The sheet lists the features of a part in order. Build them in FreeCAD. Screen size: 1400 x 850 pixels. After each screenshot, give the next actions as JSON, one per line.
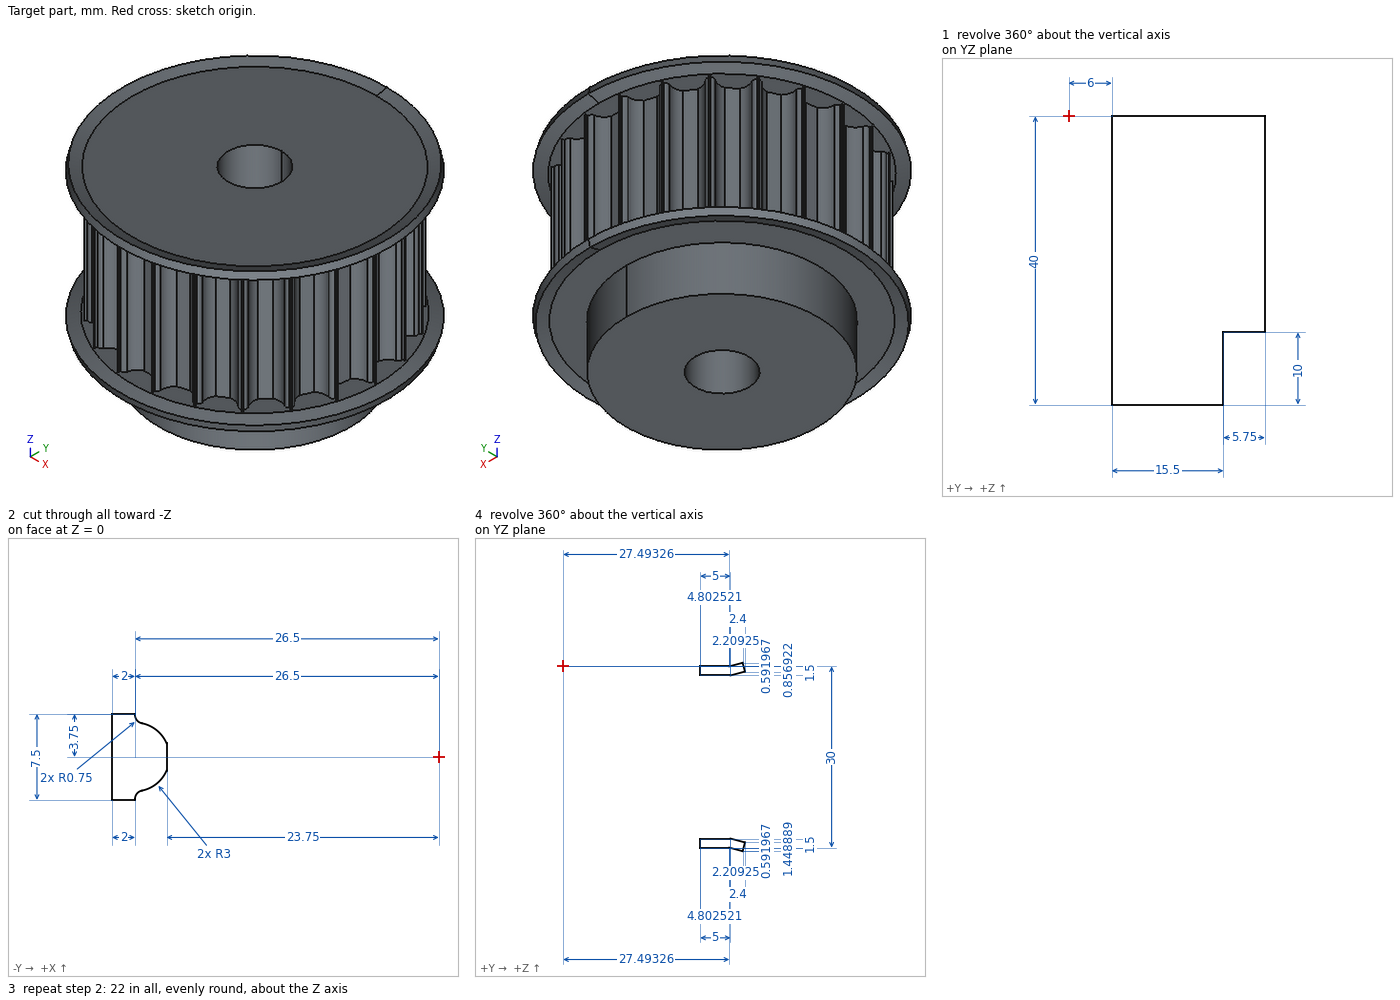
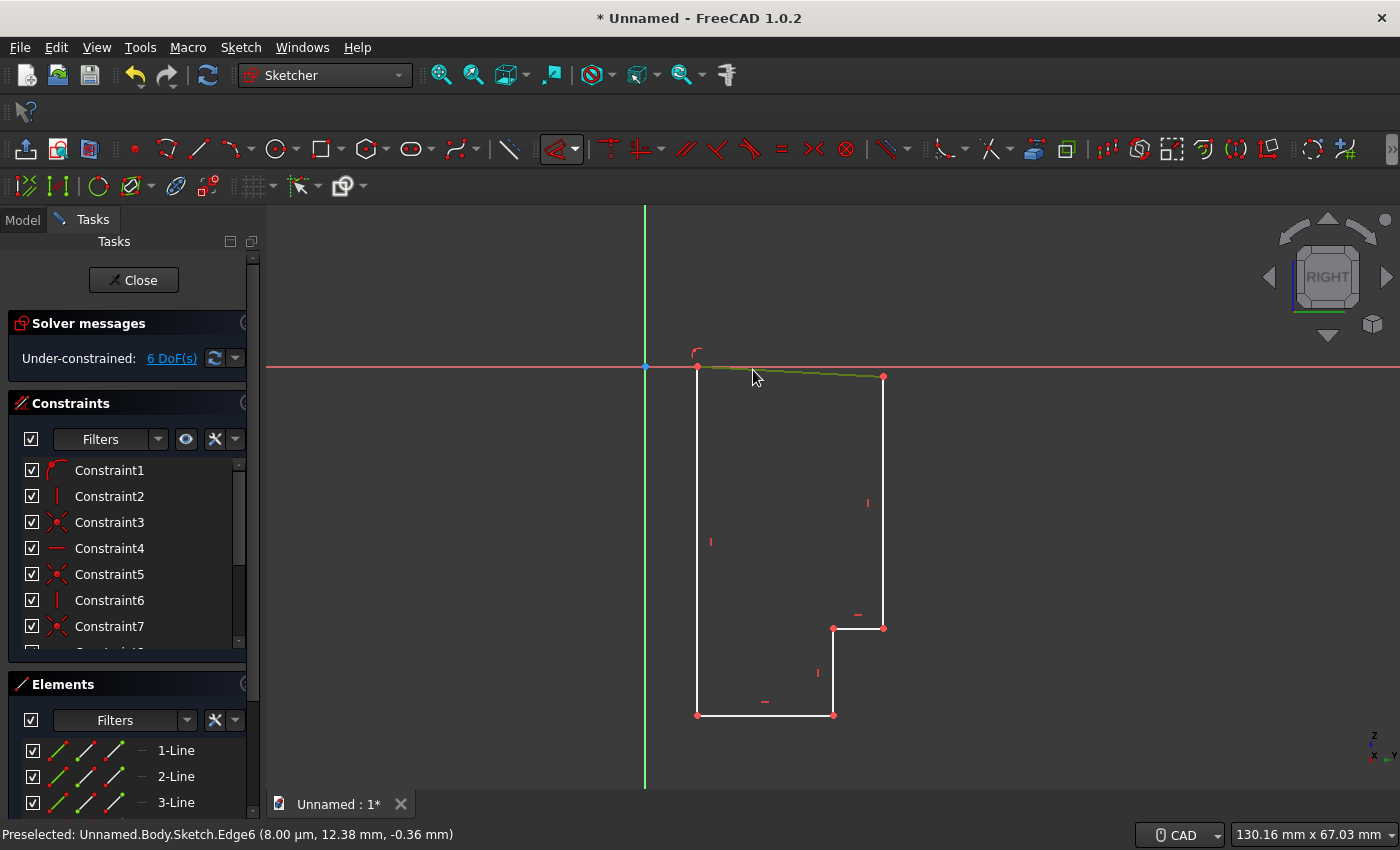
{"action": "key", "text": "h"}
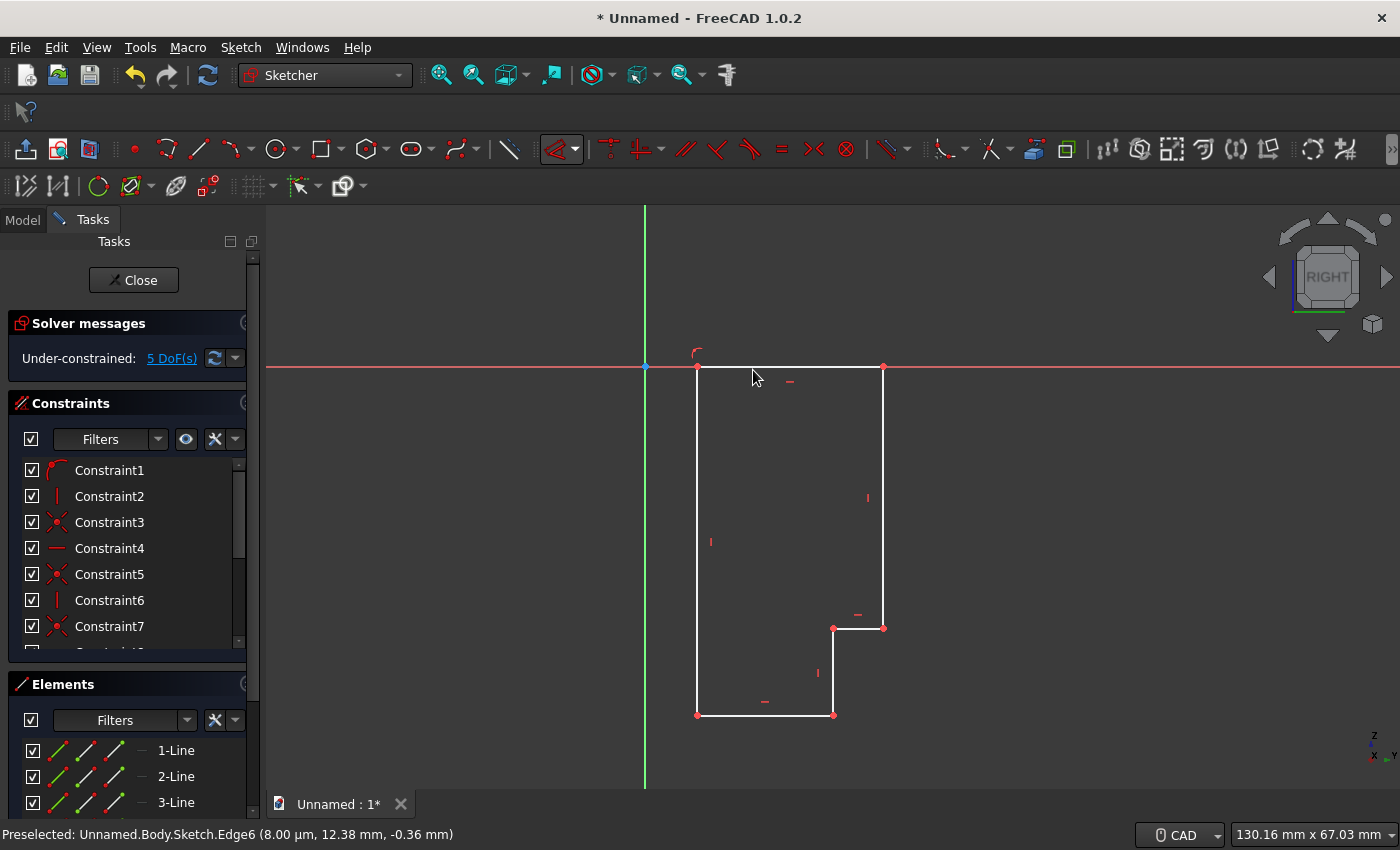
{"action": "left_click", "coordinate": [697, 471]}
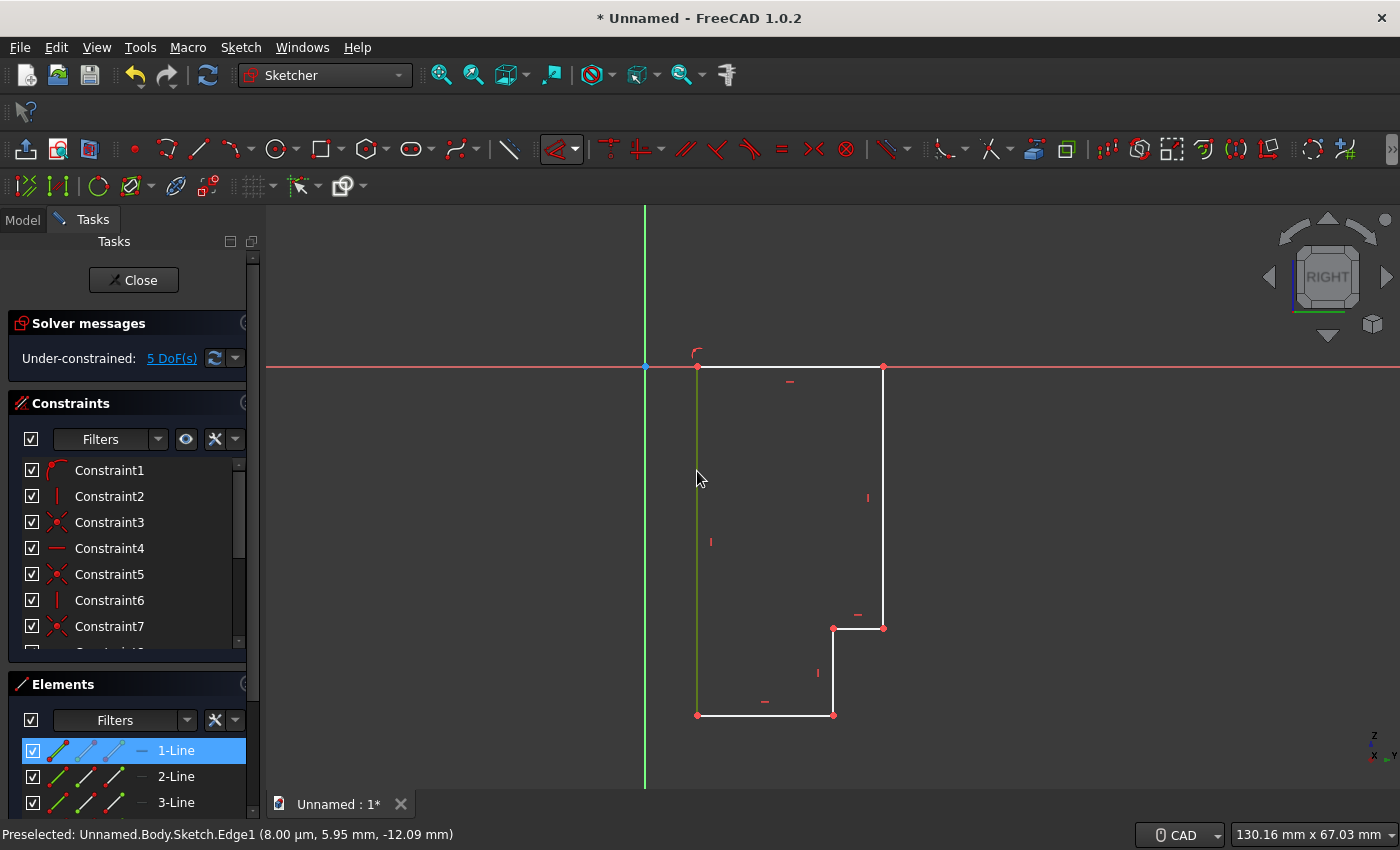
{"action": "left_click", "coordinate": [578, 150]}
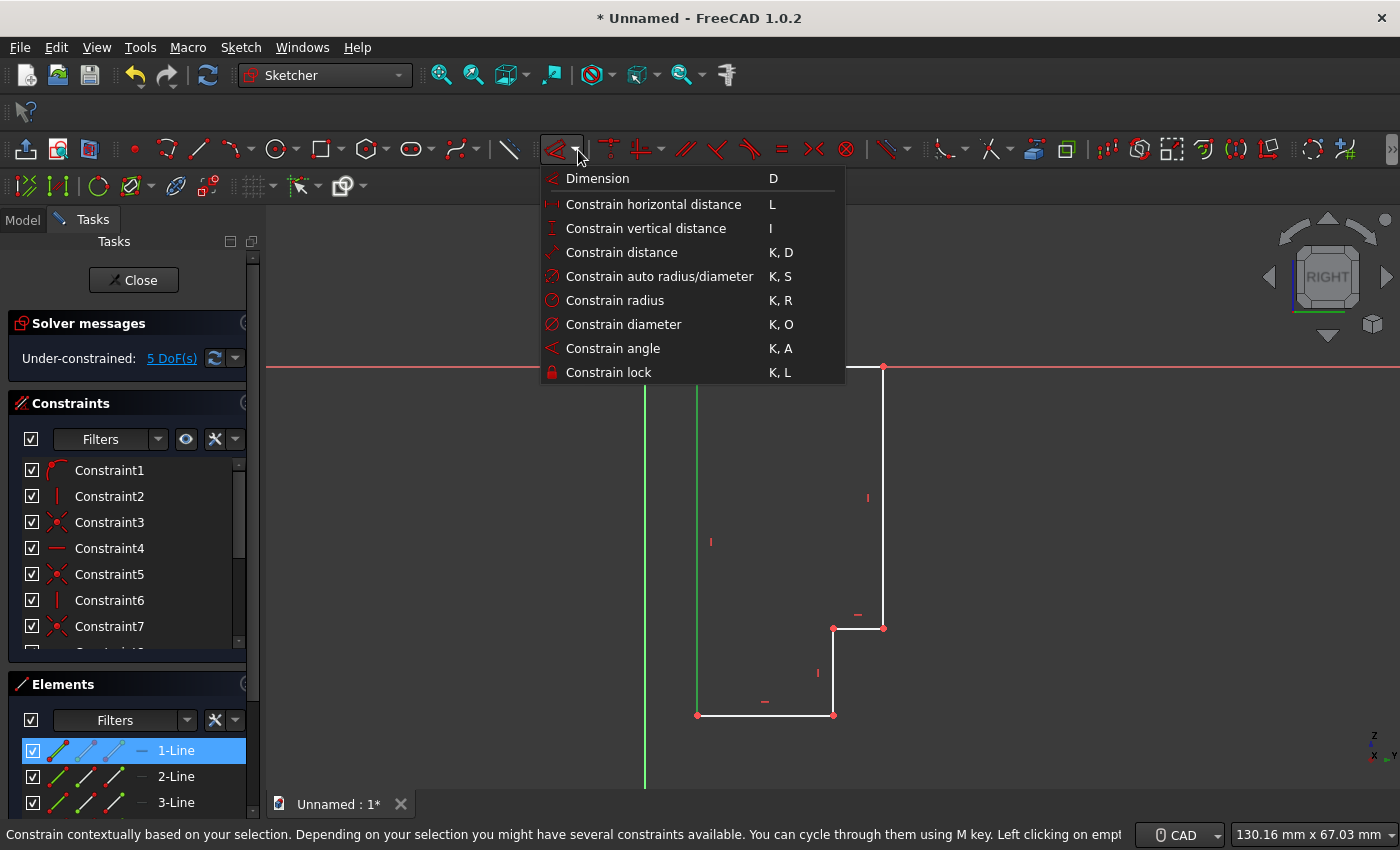
{"action": "left_click", "coordinate": [693, 228]}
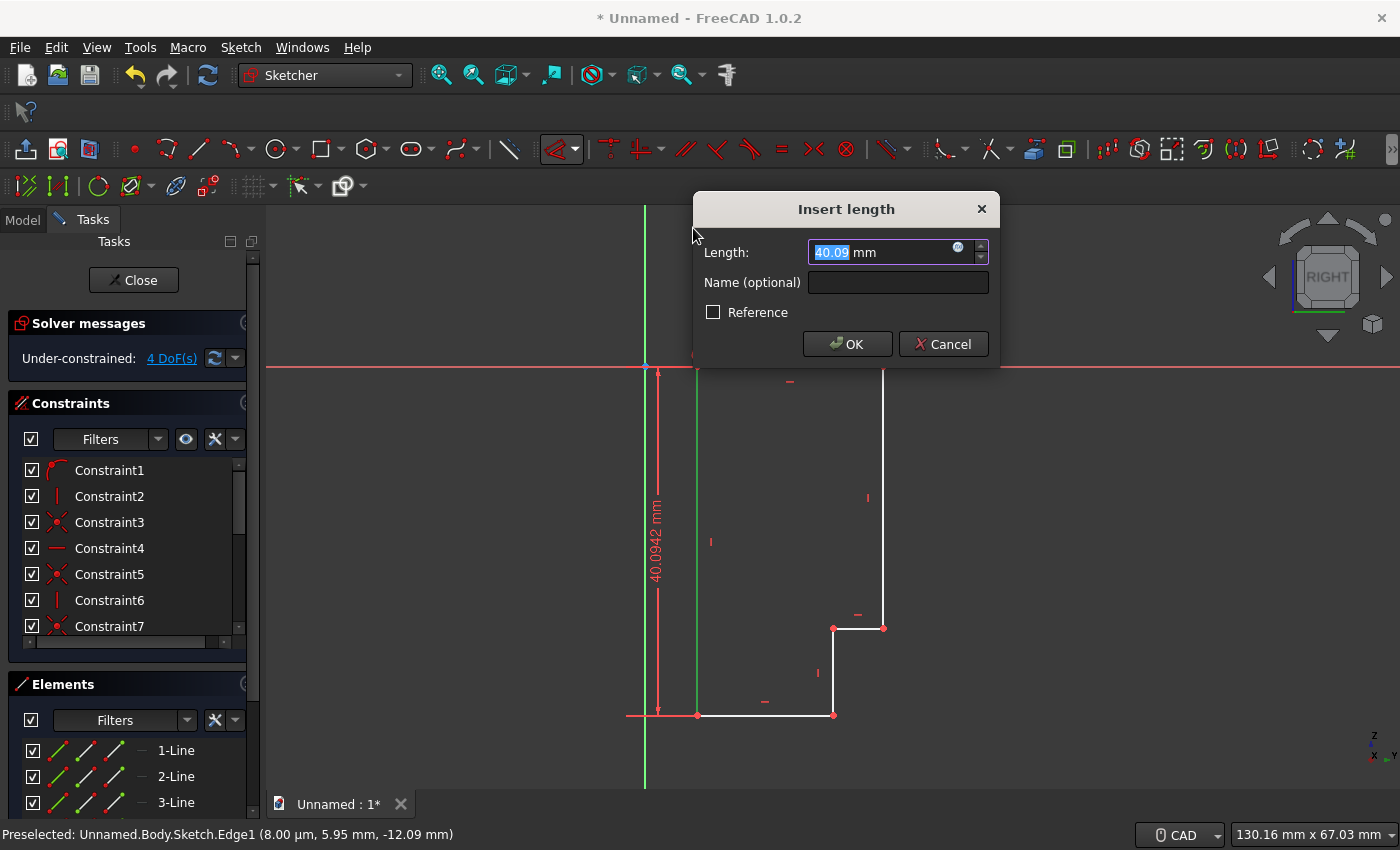
{"action": "type", "text": "40"}
{"action": "key", "text": "Return"}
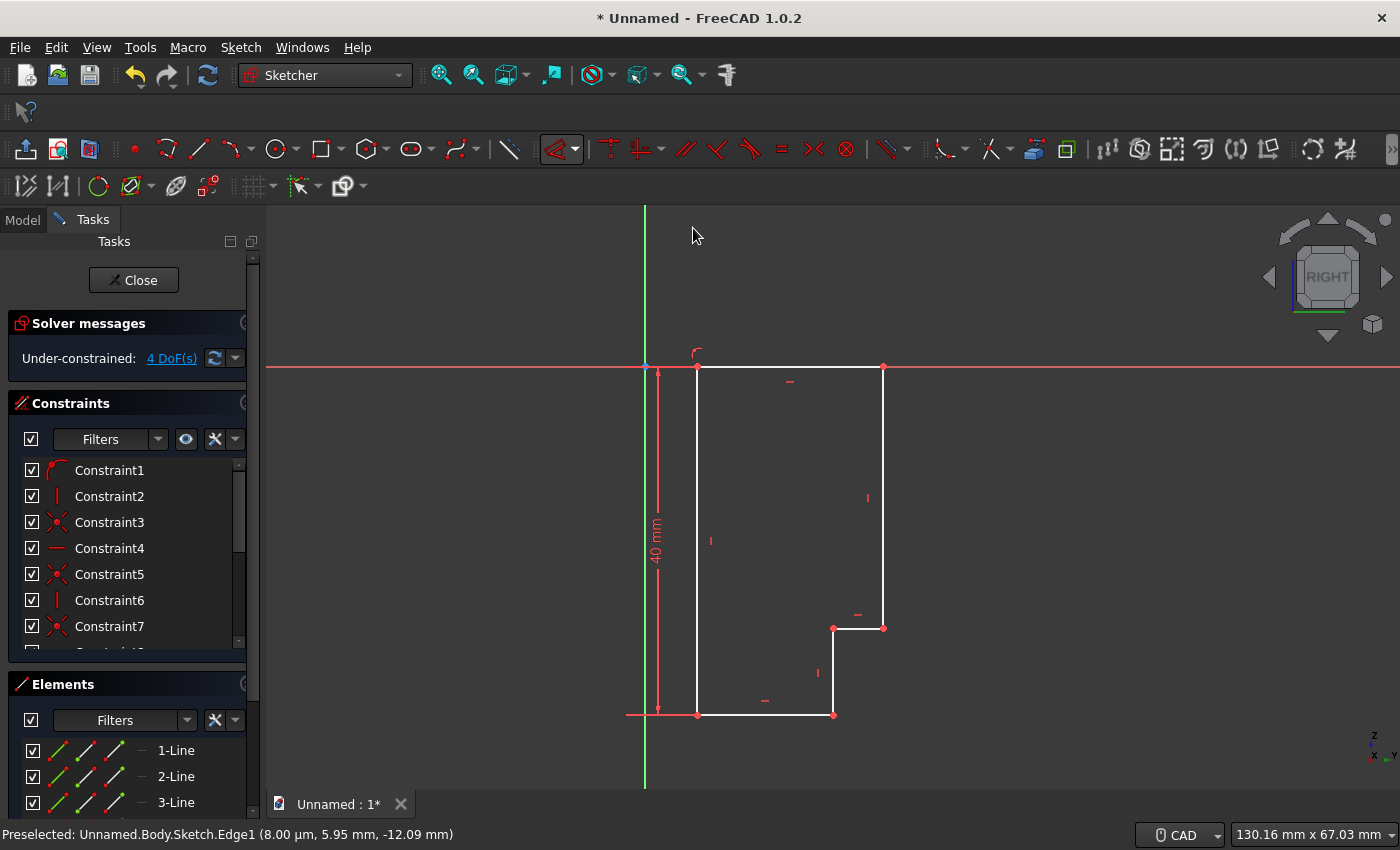
{"action": "left_click", "coordinate": [833, 689]}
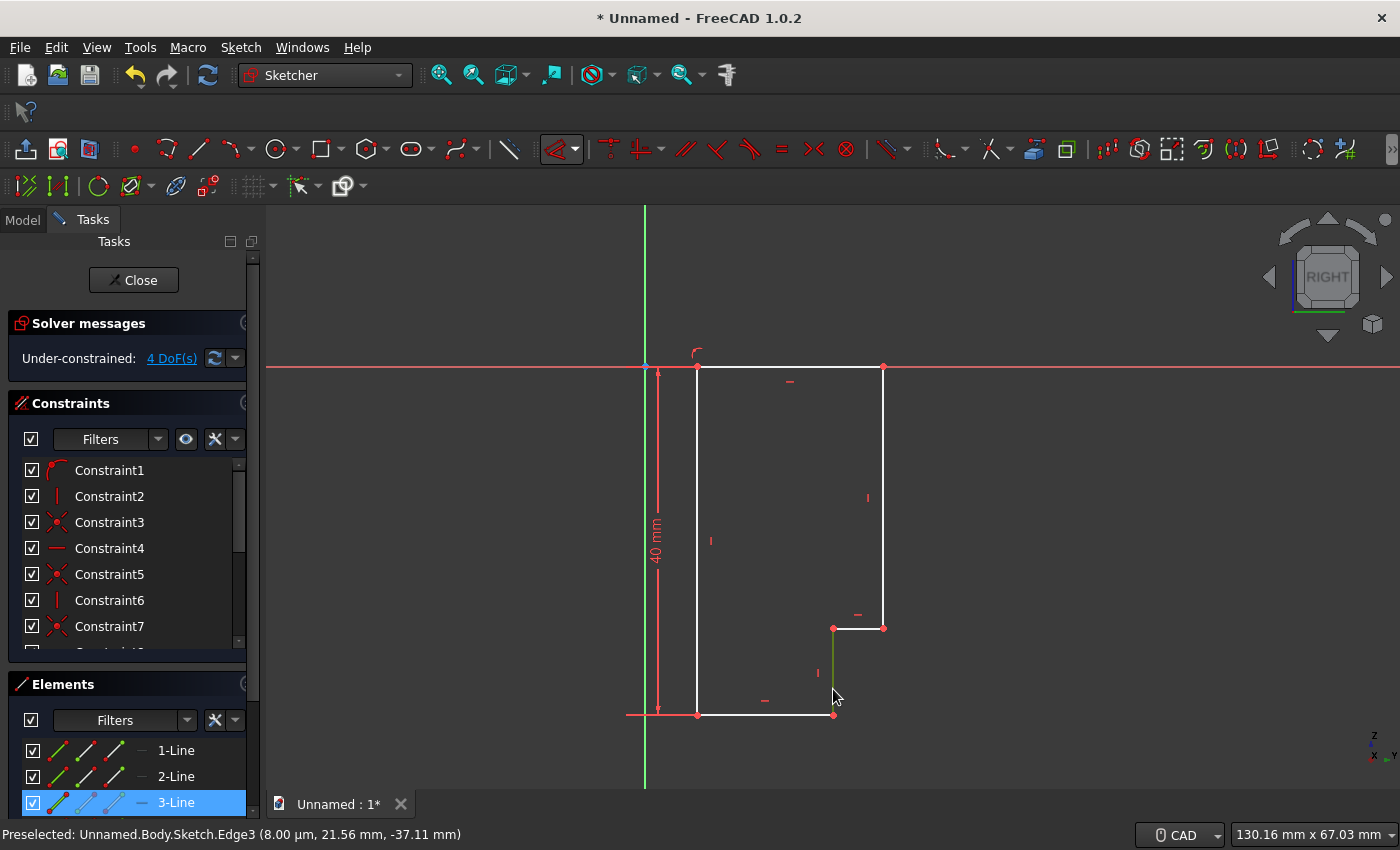
{"action": "key", "text": "i"}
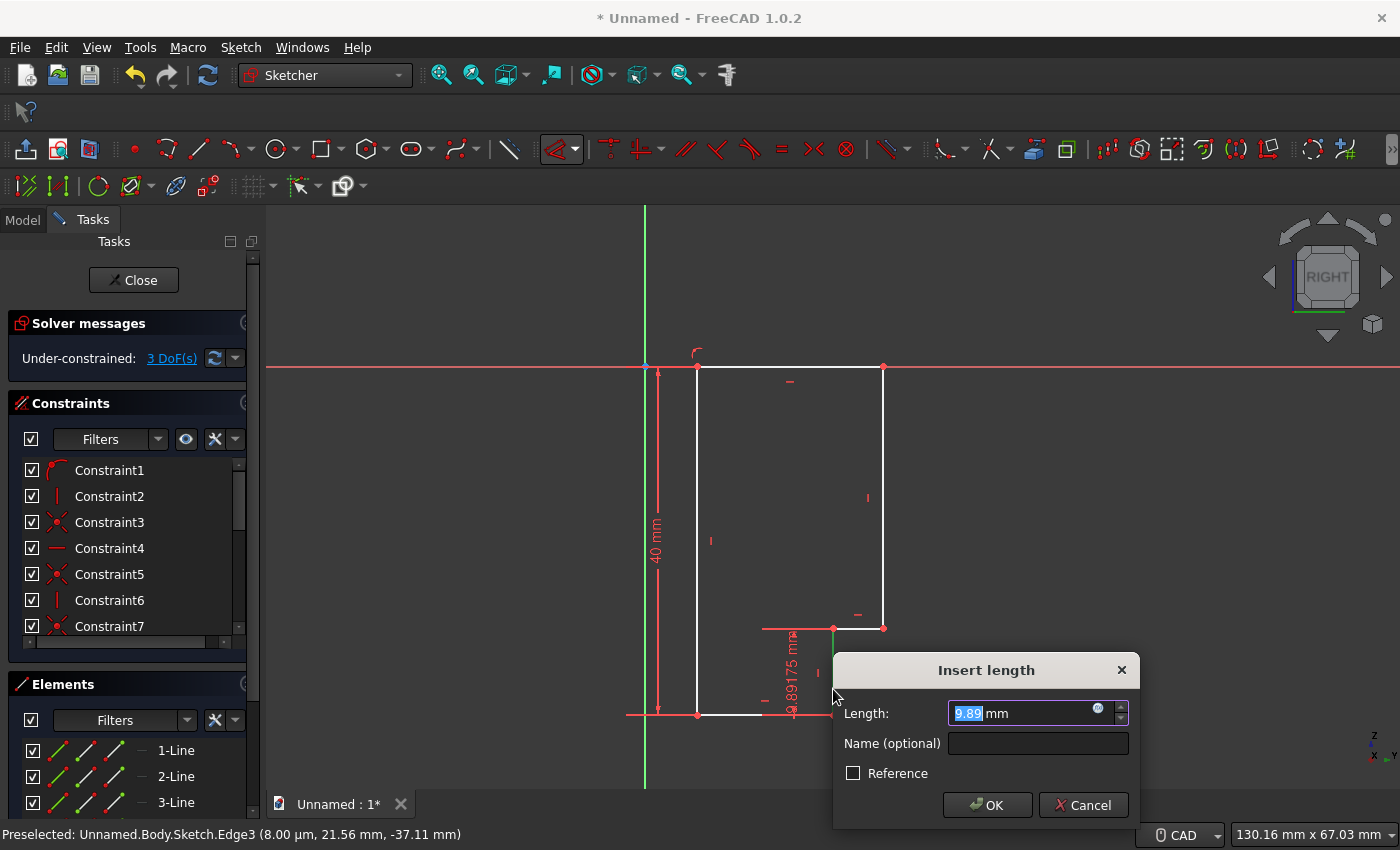
{"action": "type", "text": "10"}
{"action": "key", "text": "Return"}